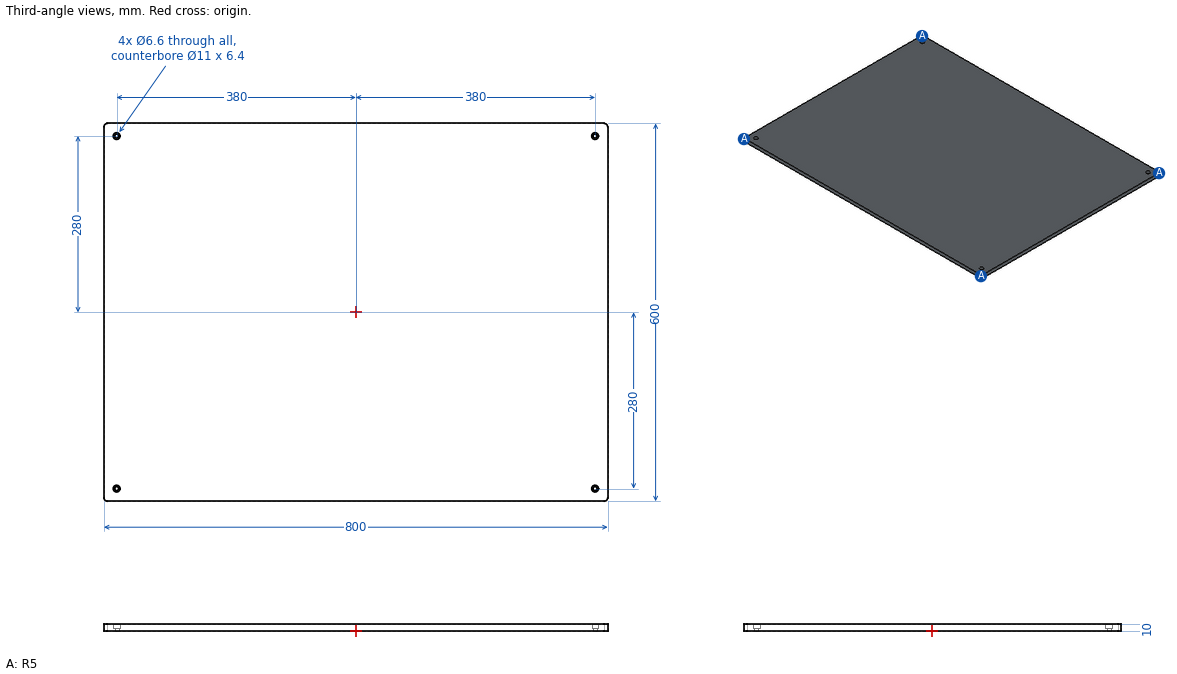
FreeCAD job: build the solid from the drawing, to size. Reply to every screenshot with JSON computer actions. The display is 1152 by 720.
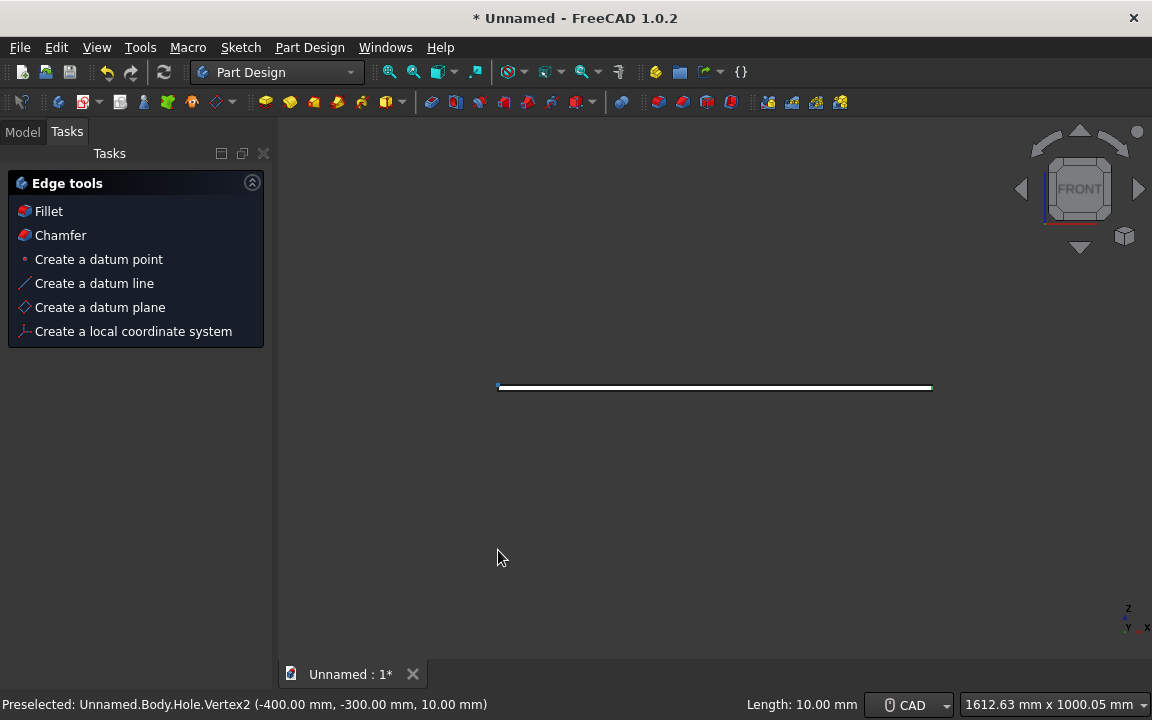
{"action": "scroll", "coordinate": [498, 387], "scroll_direction": "up", "scroll_amount": 10}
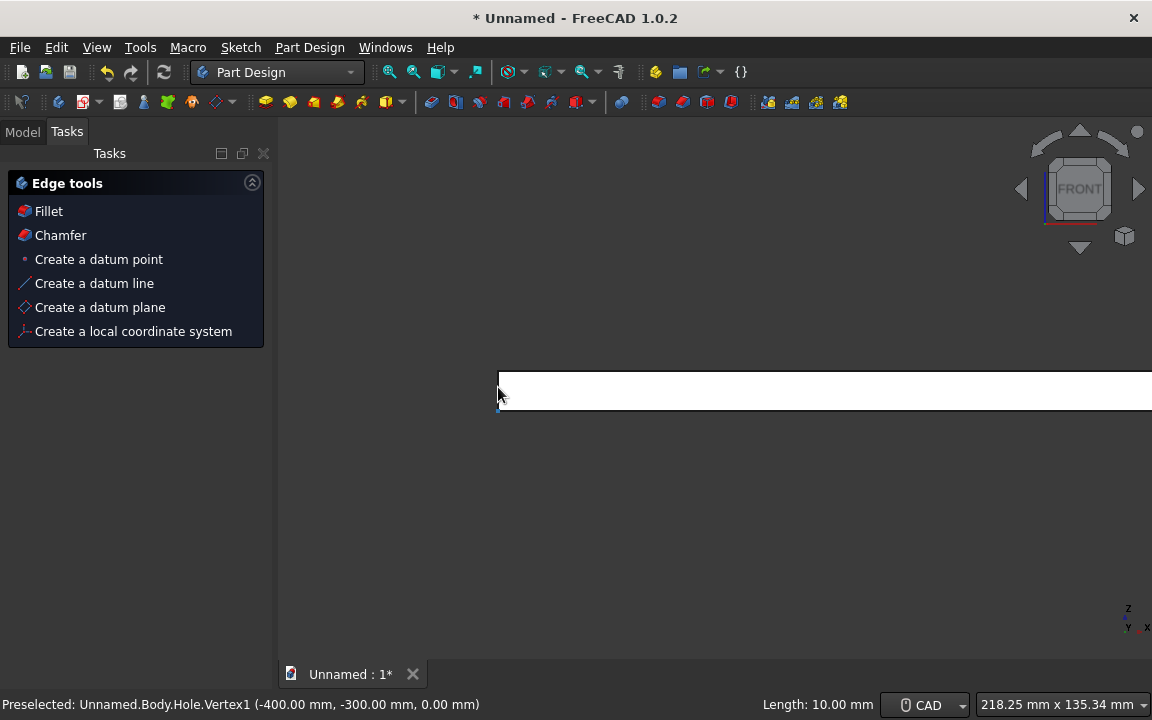
{"action": "left_click", "coordinate": [498, 390], "text": "ctrl"}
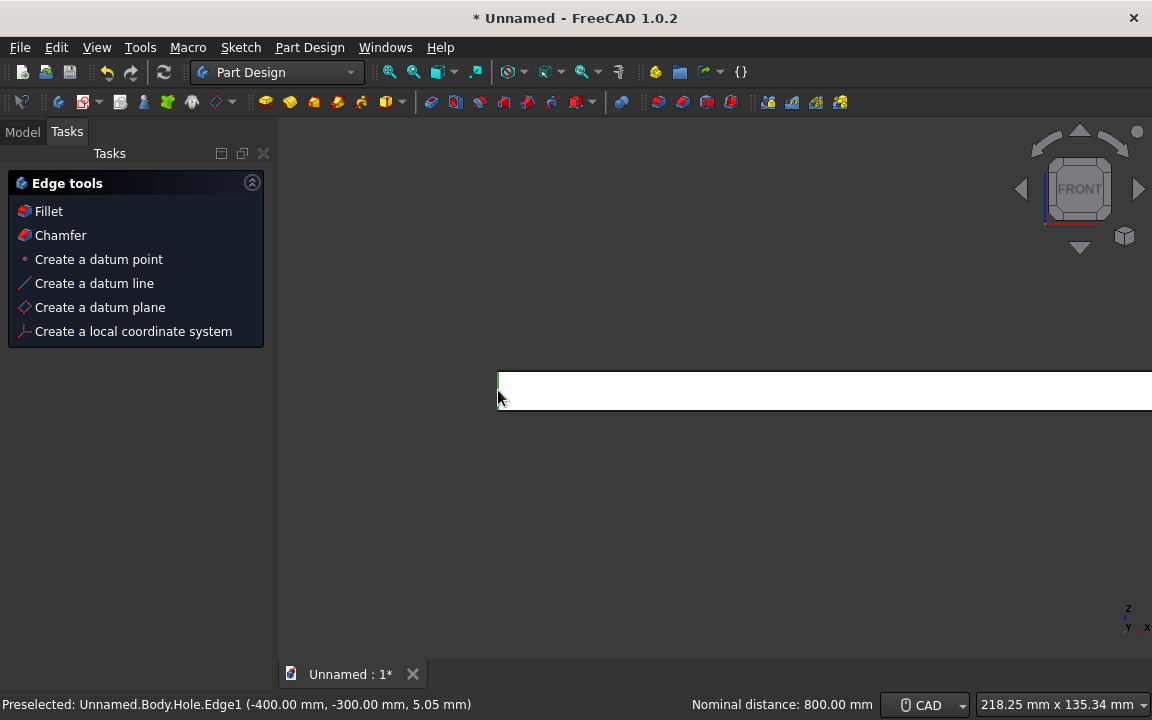
{"action": "left_click", "coordinate": [390, 72]}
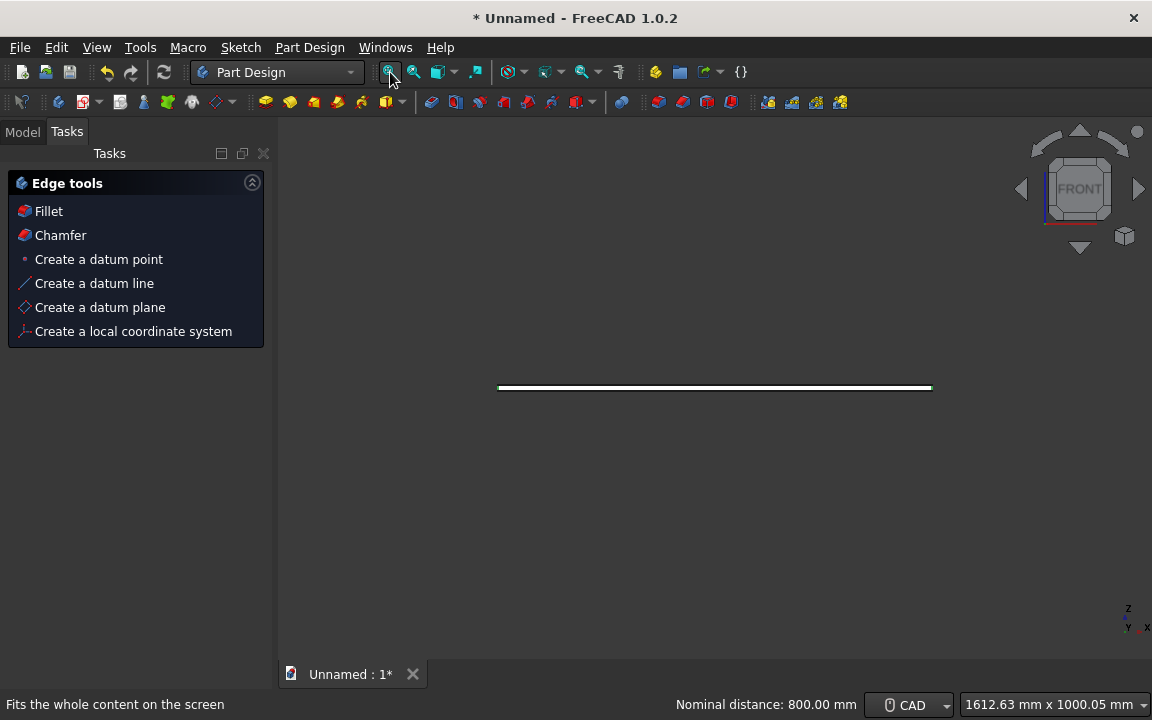
{"action": "key", "text": "3"}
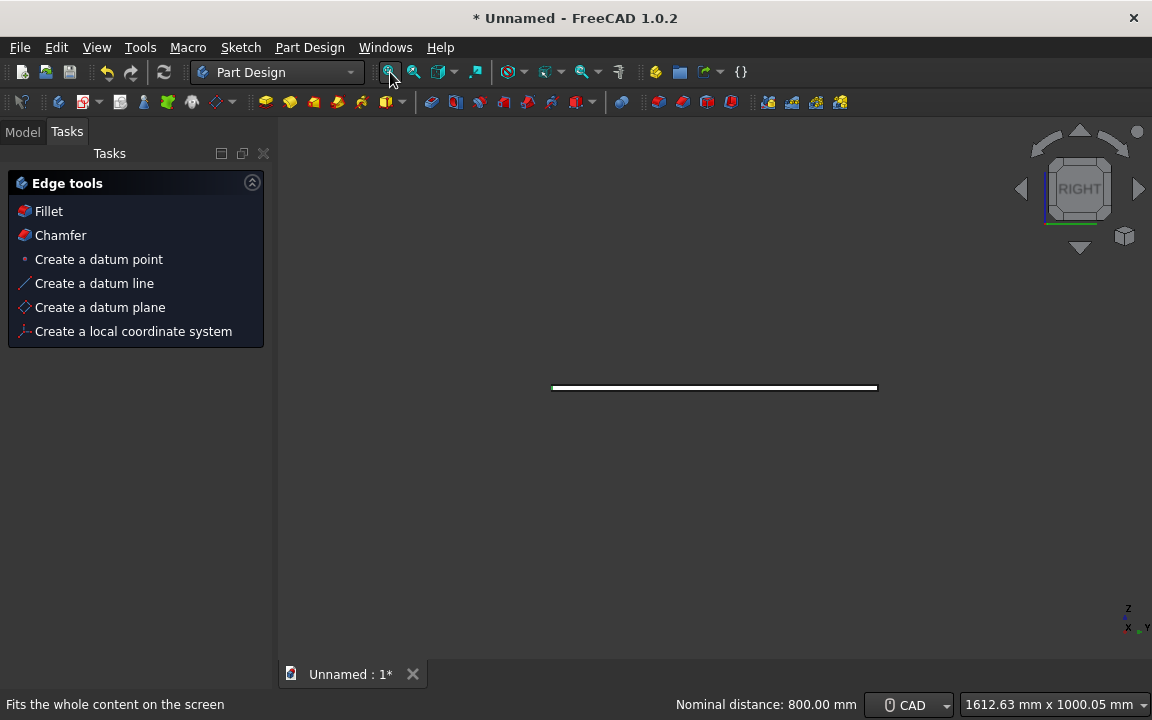
{"action": "key", "text": "v f"}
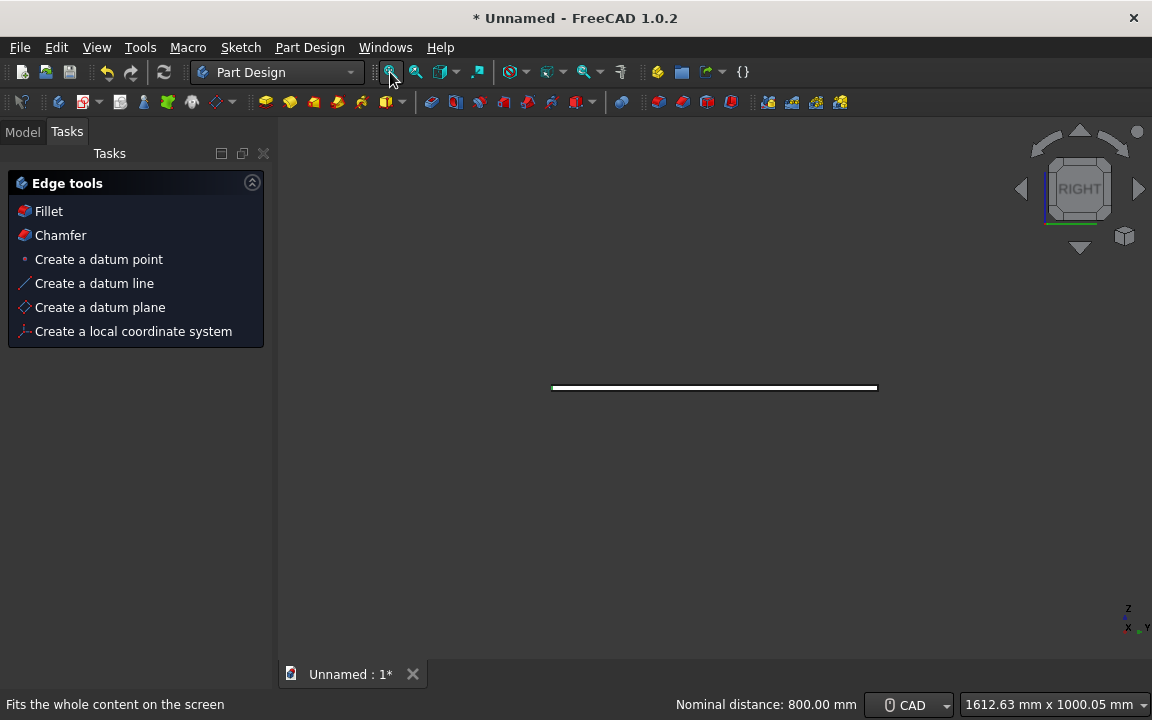
{"action": "scroll", "coordinate": [878, 387], "scroll_direction": "up", "scroll_amount": 10}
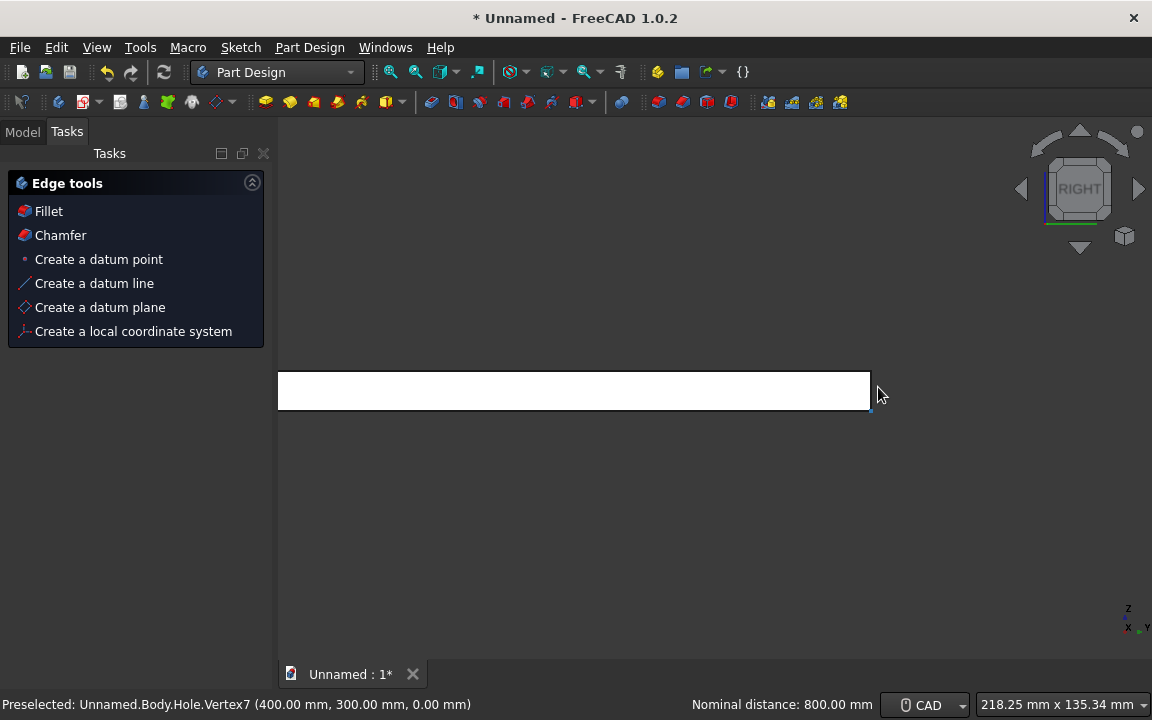
{"action": "left_click", "coordinate": [871, 390], "text": "ctrl"}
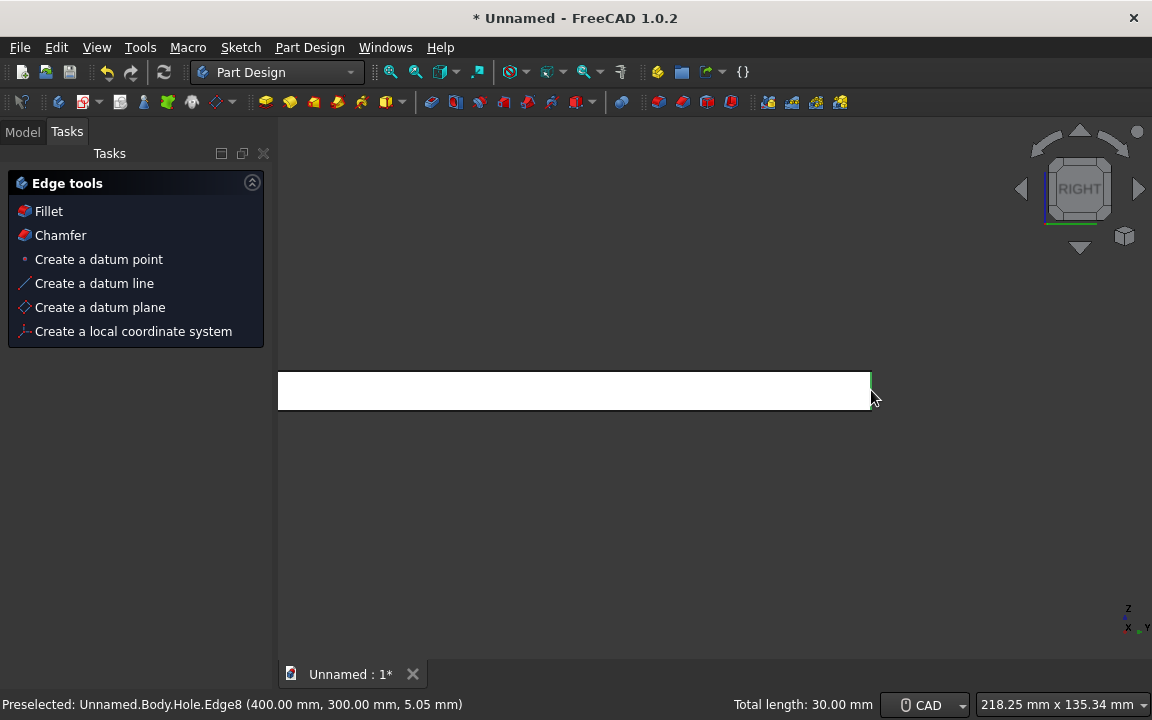
{"action": "left_click", "coordinate": [392, 72]}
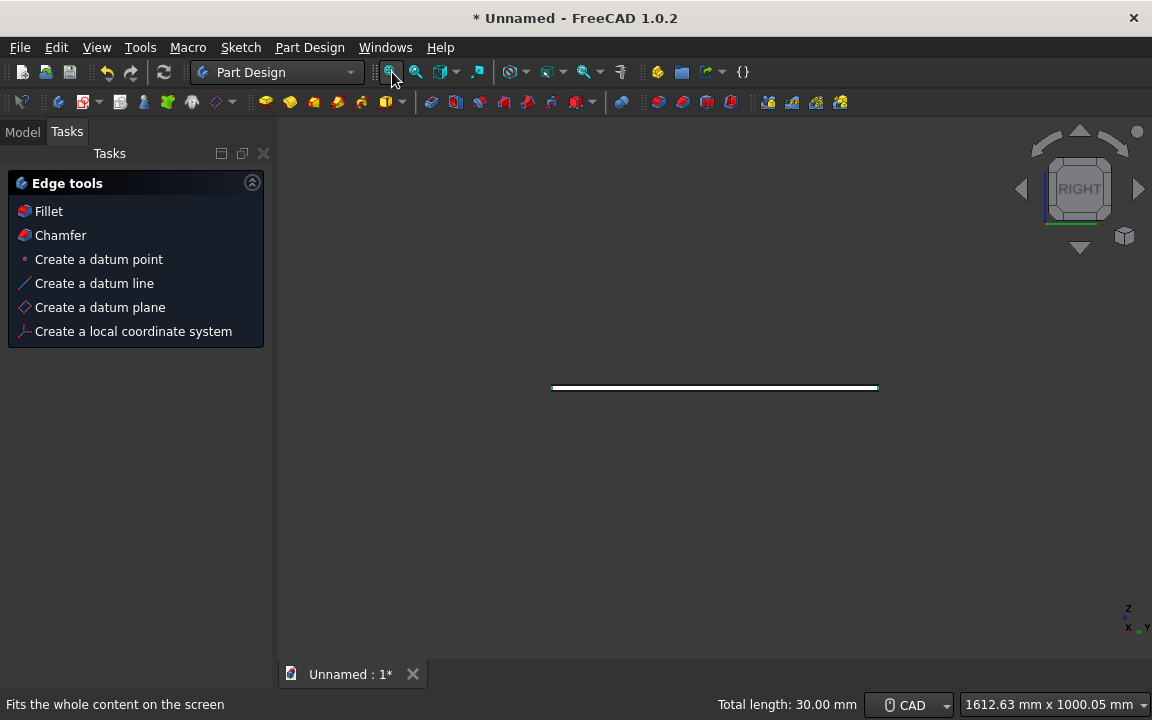
{"action": "key", "text": "5"}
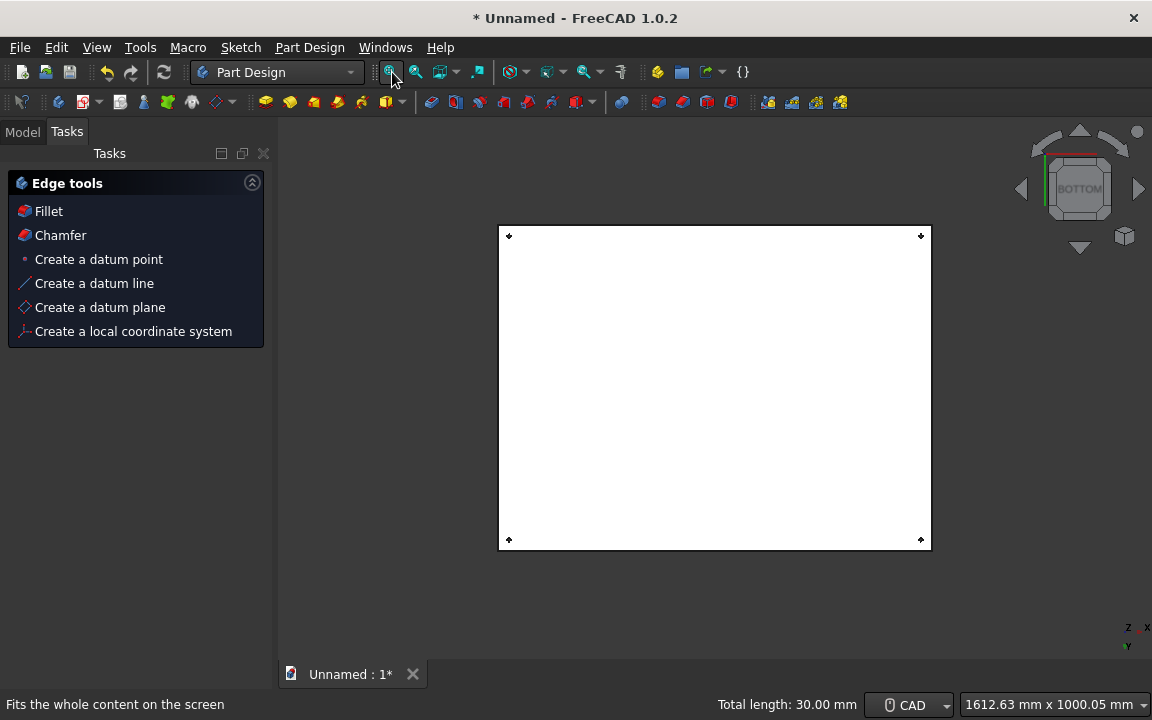
{"action": "scroll", "coordinate": [498, 550], "scroll_direction": "up", "scroll_amount": 10}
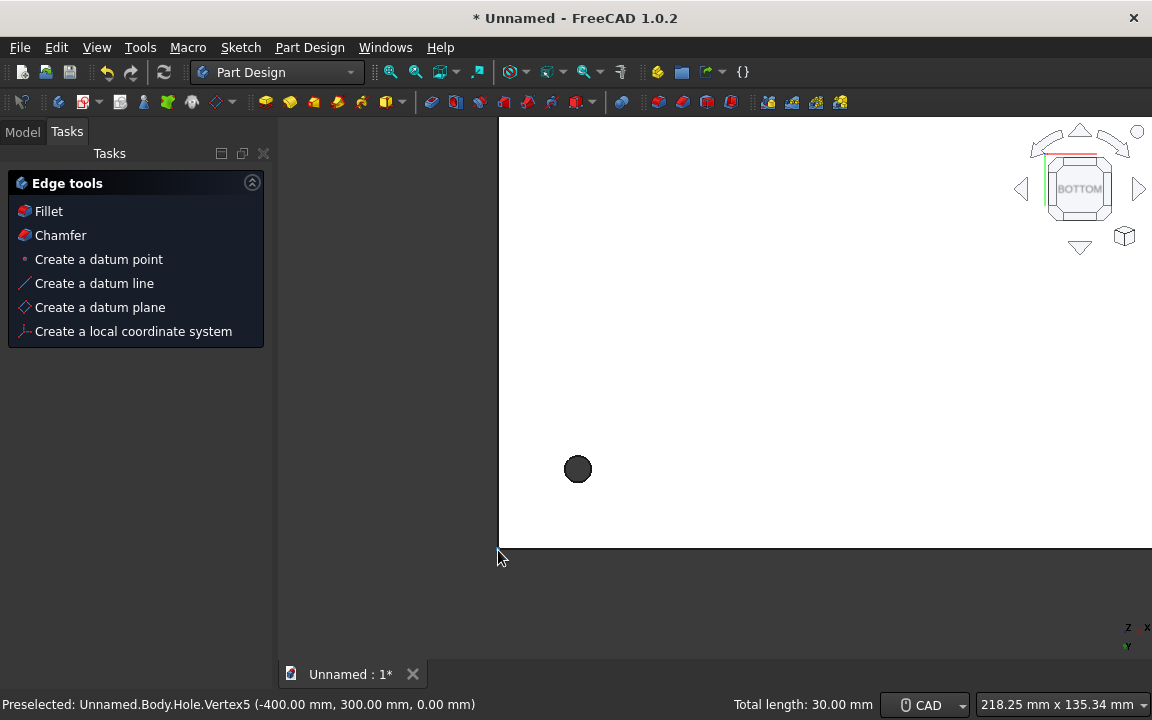
{"action": "left_click", "coordinate": [392, 72]}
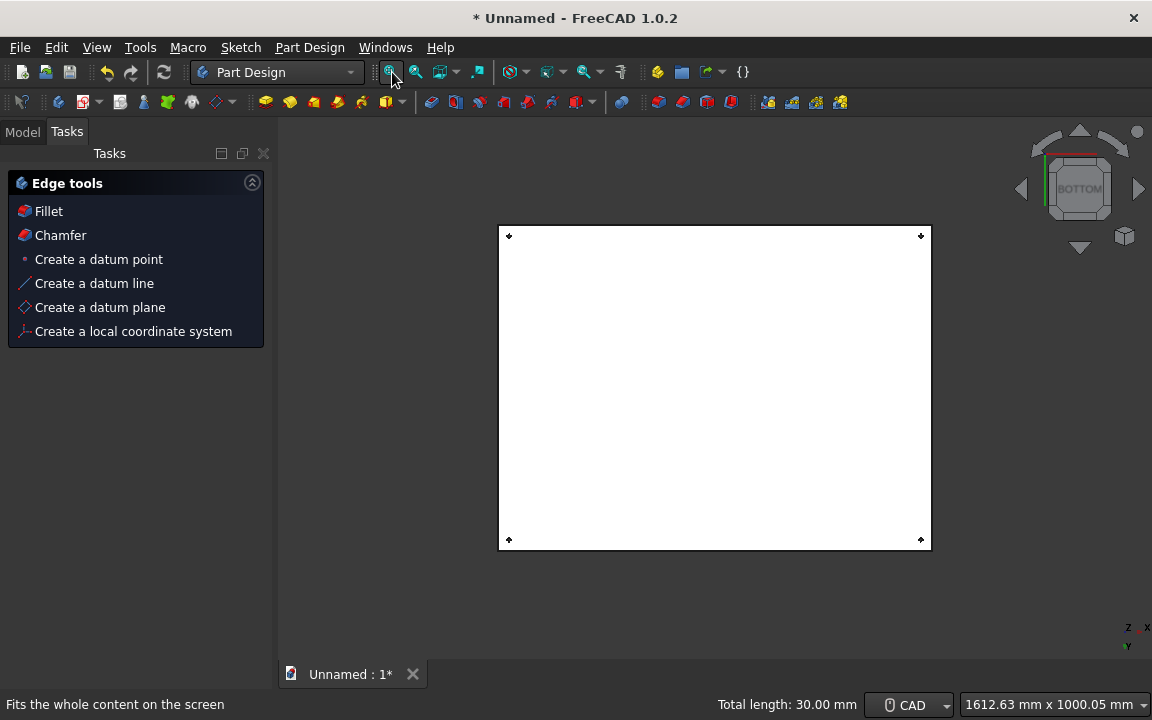
{"action": "key", "text": "4"}